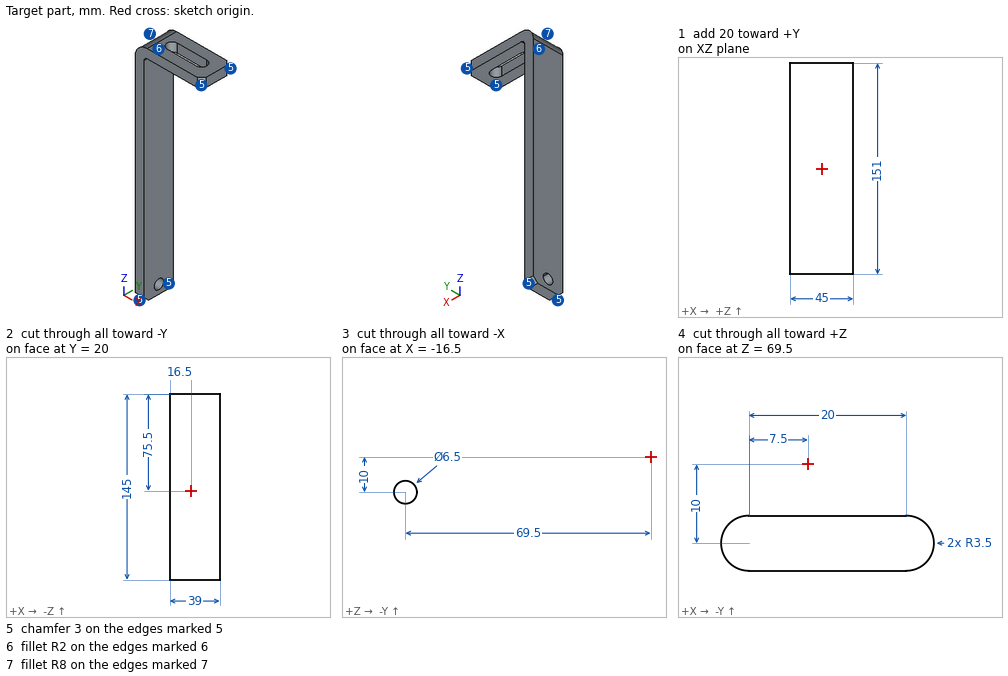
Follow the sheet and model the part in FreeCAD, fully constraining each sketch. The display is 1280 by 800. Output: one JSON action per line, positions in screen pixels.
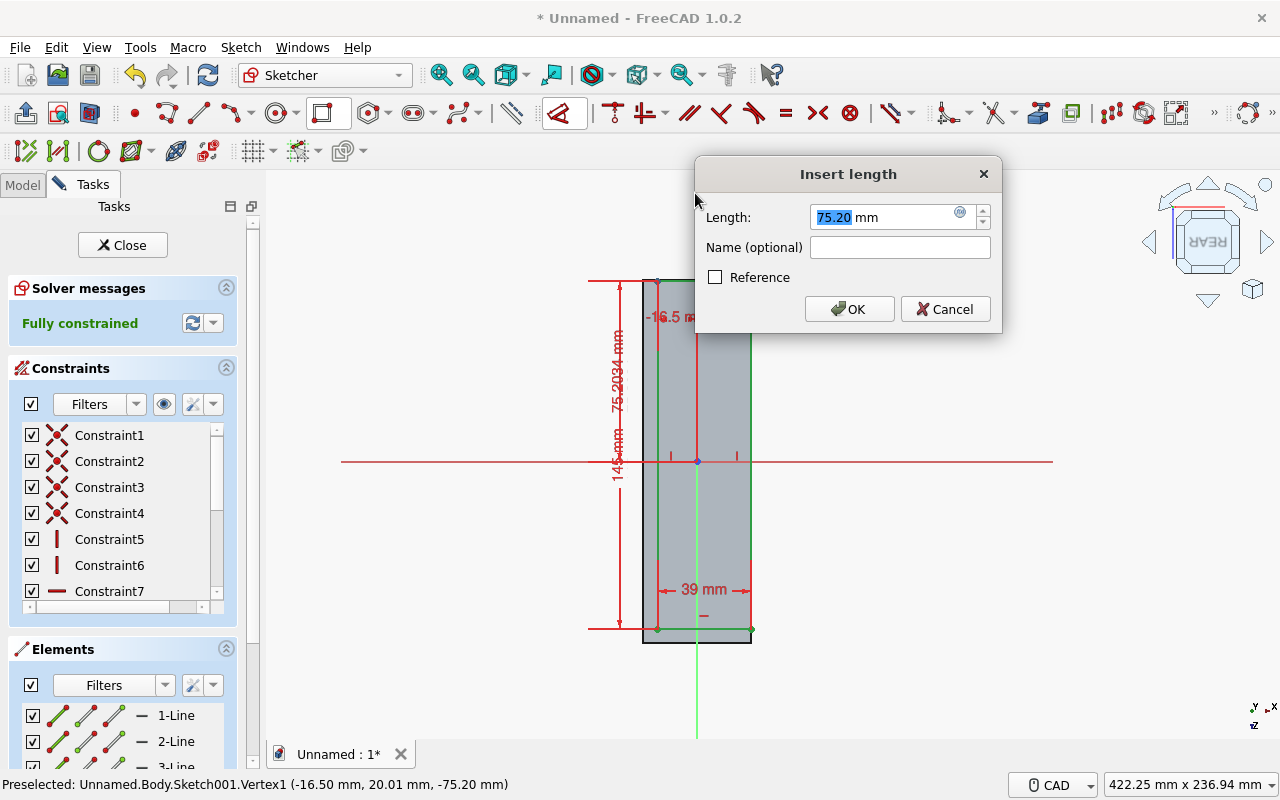
{"action": "type", "text": "75.5"}
{"action": "key", "text": "Return"}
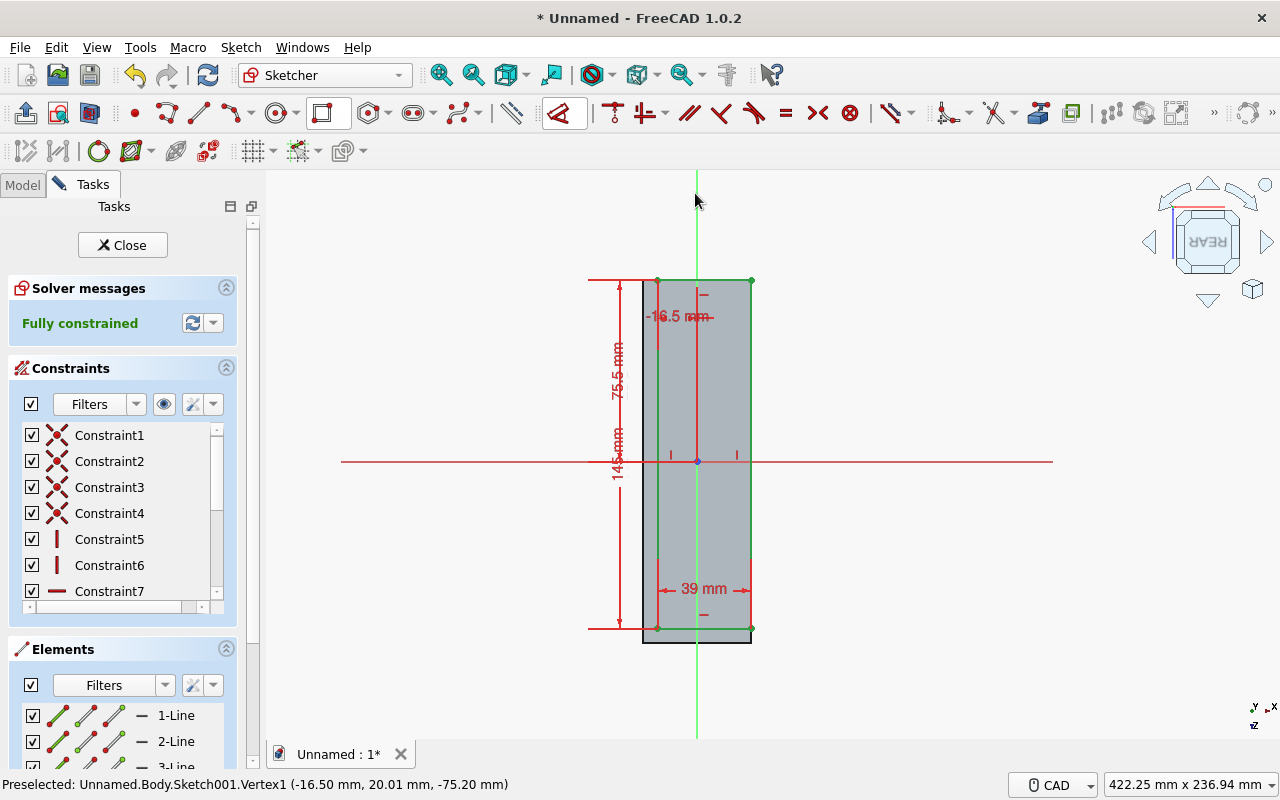
{"action": "left_click", "coordinate": [123, 245]}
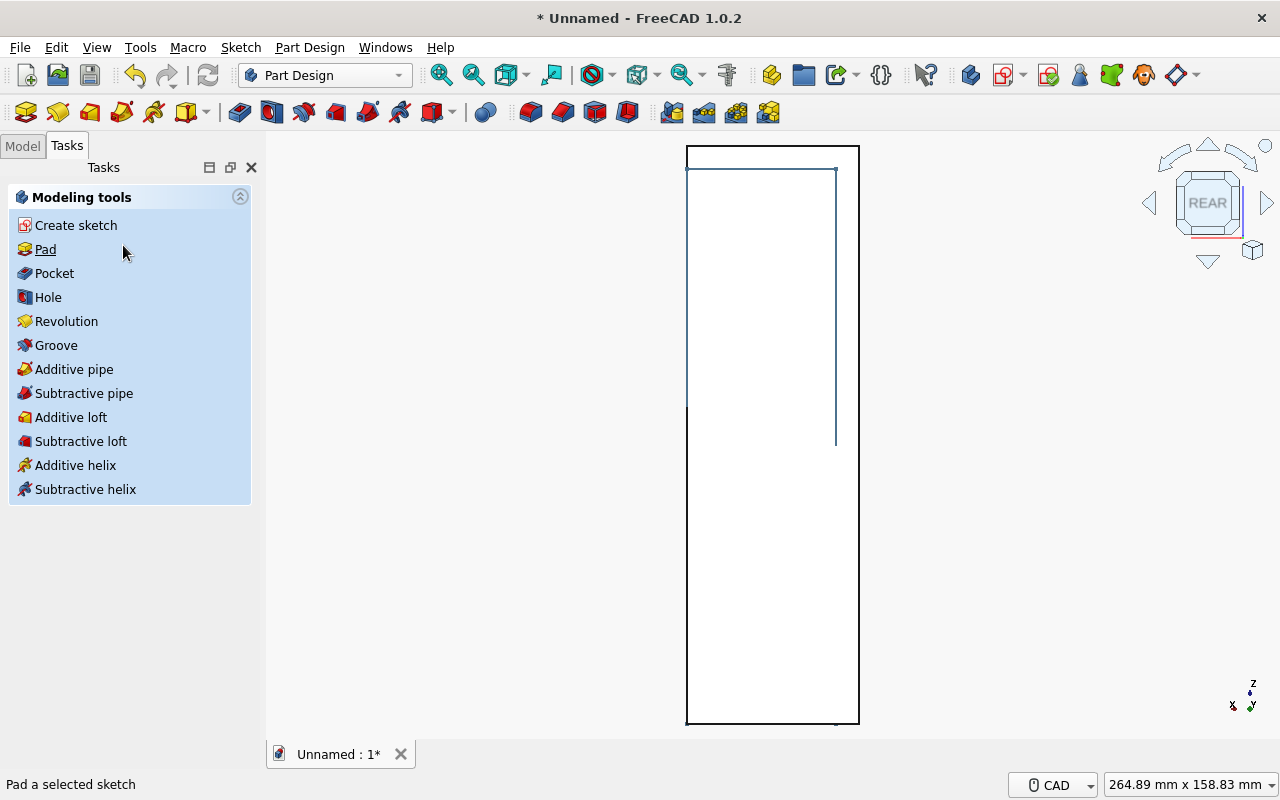
{"action": "left_click", "coordinate": [240, 112]}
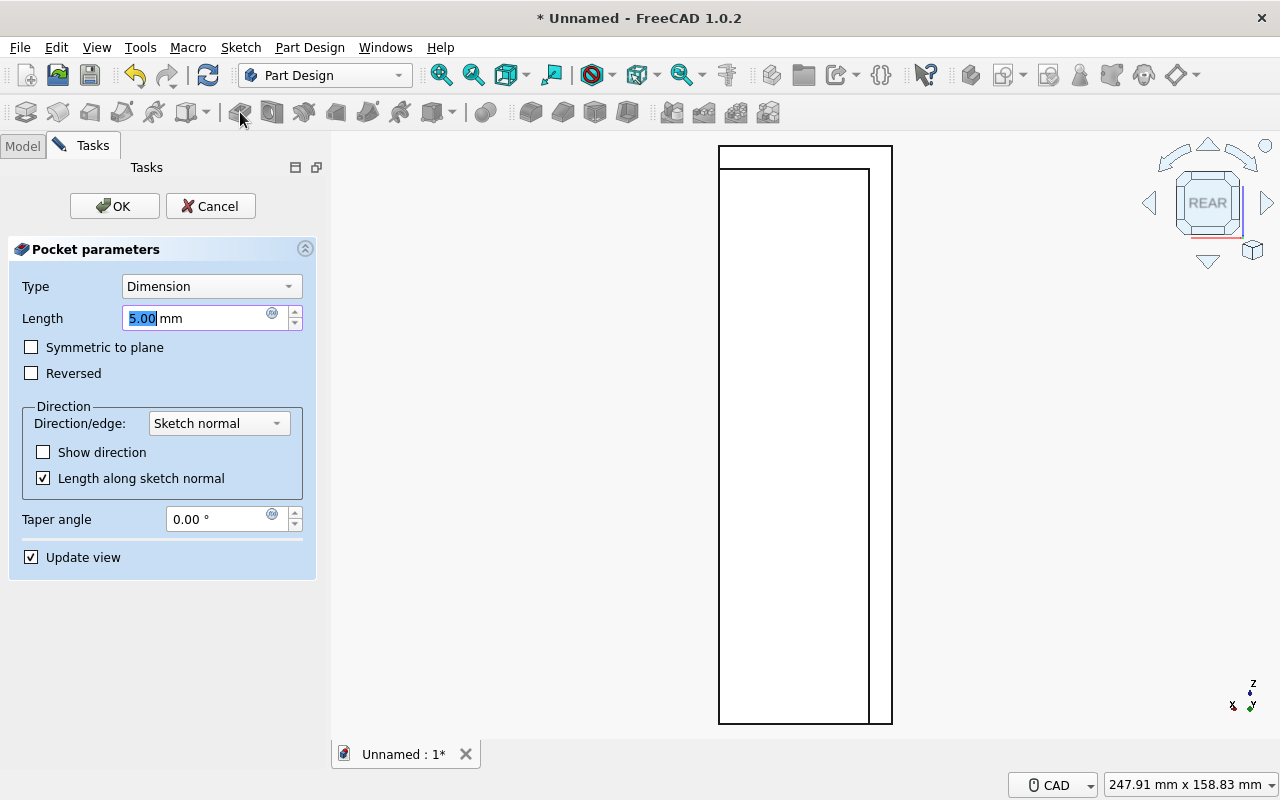
{"action": "left_click", "coordinate": [212, 286]}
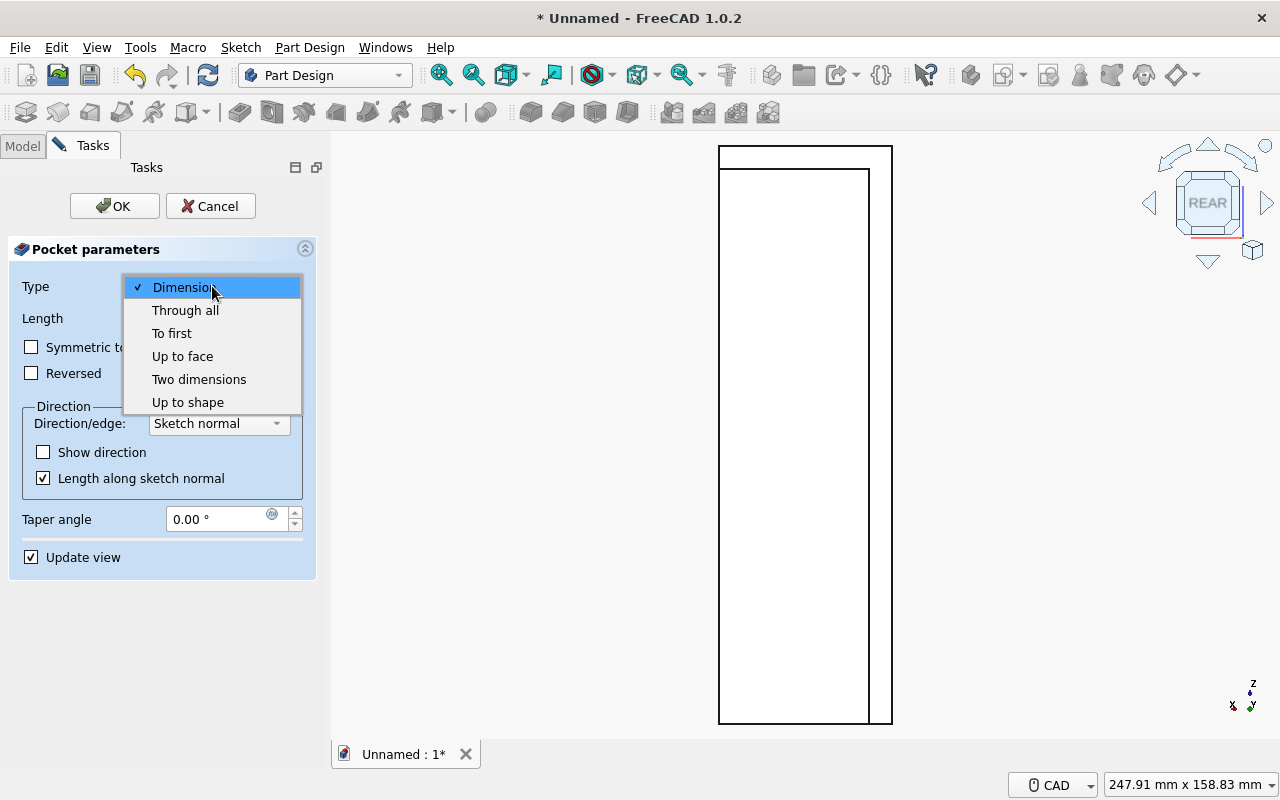
{"action": "left_click", "coordinate": [212, 310]}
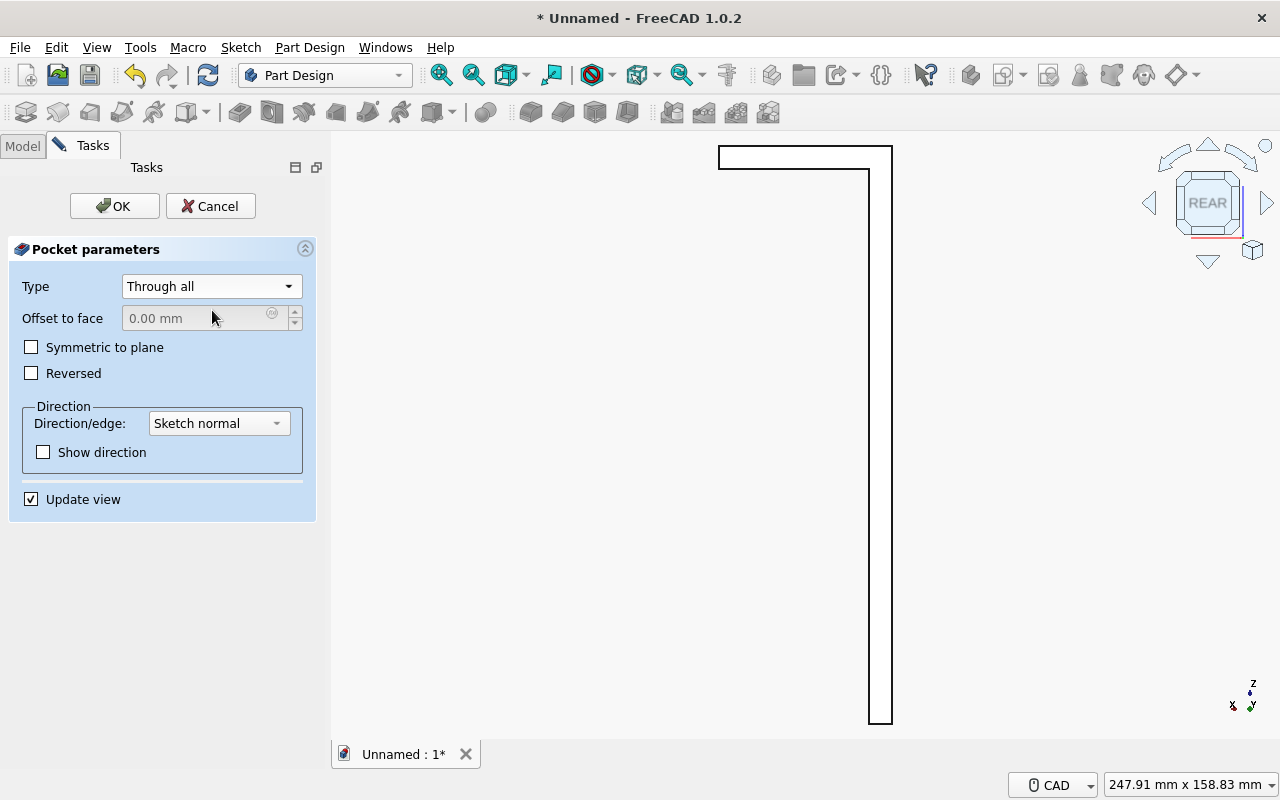
{"action": "left_click", "coordinate": [115, 206]}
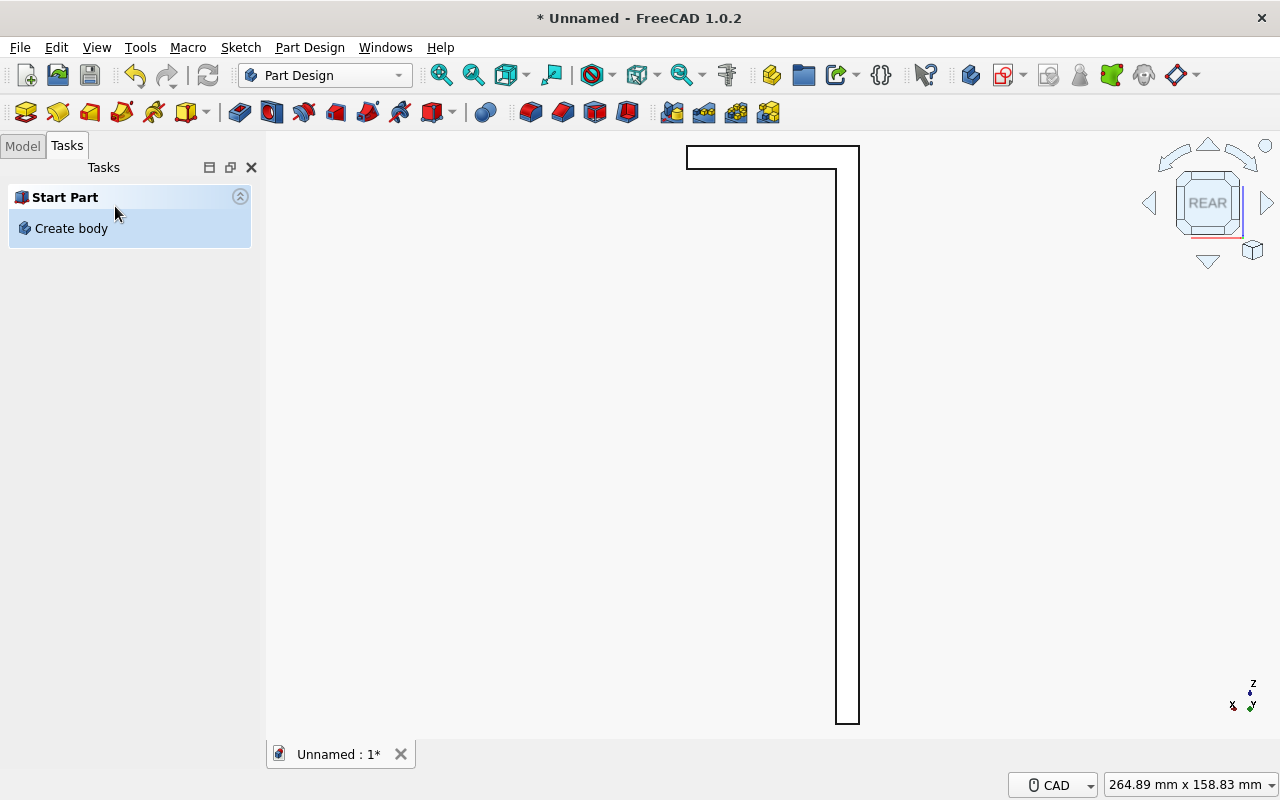
{"action": "key", "text": "0"}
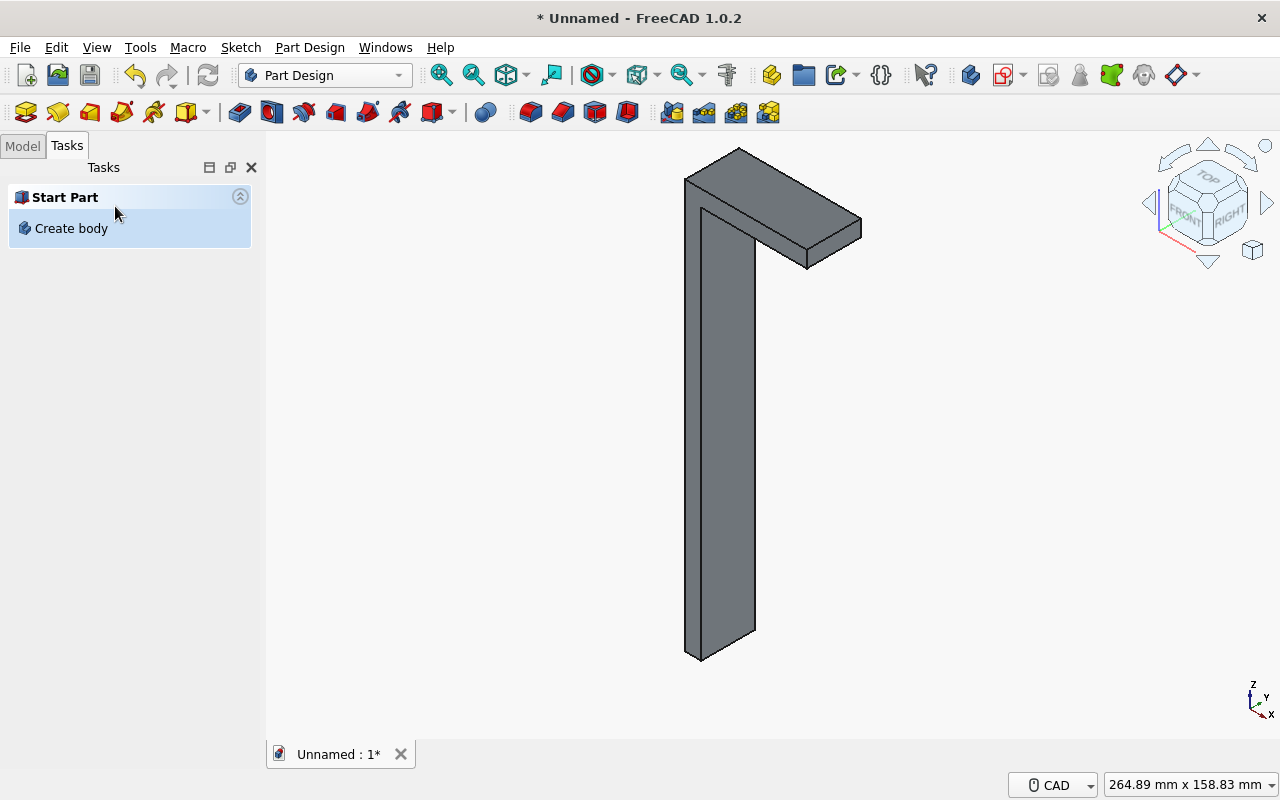
{"action": "left_click", "coordinate": [728, 612]}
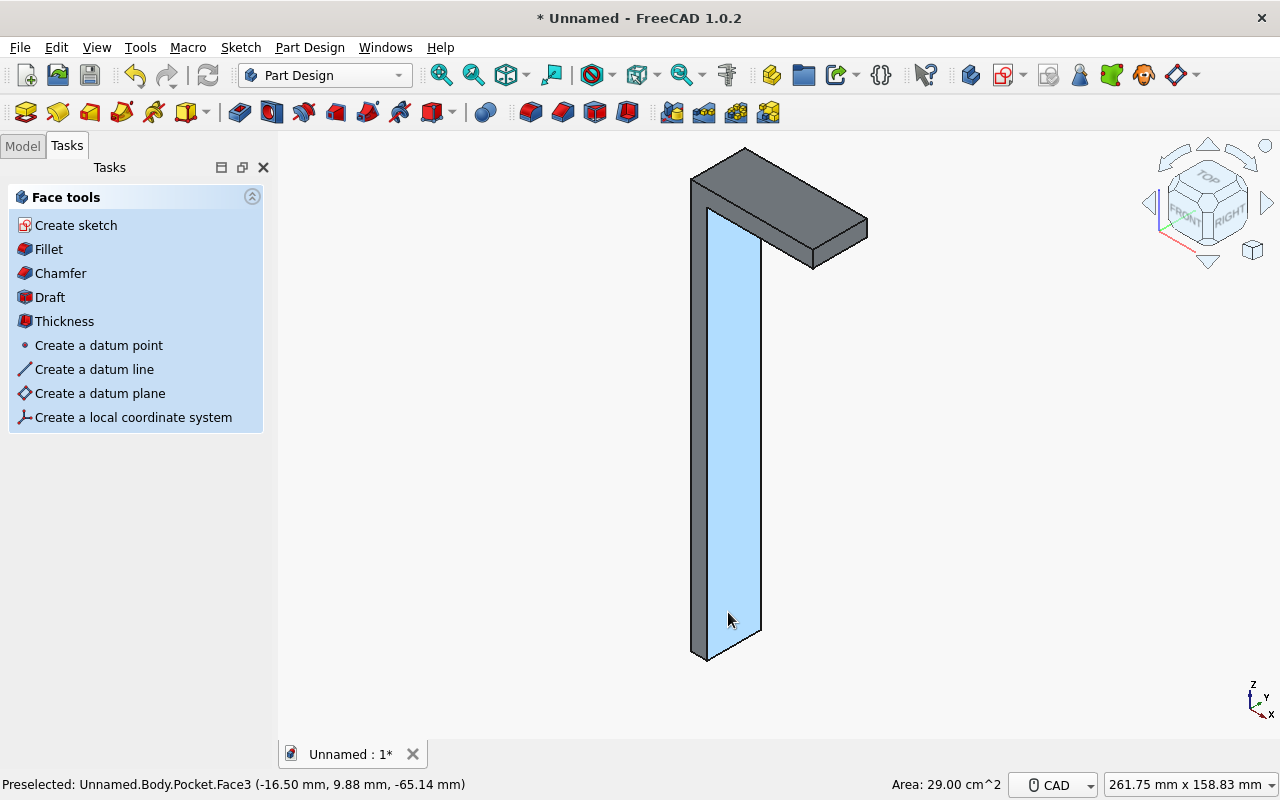
{"action": "left_click", "coordinate": [1004, 76]}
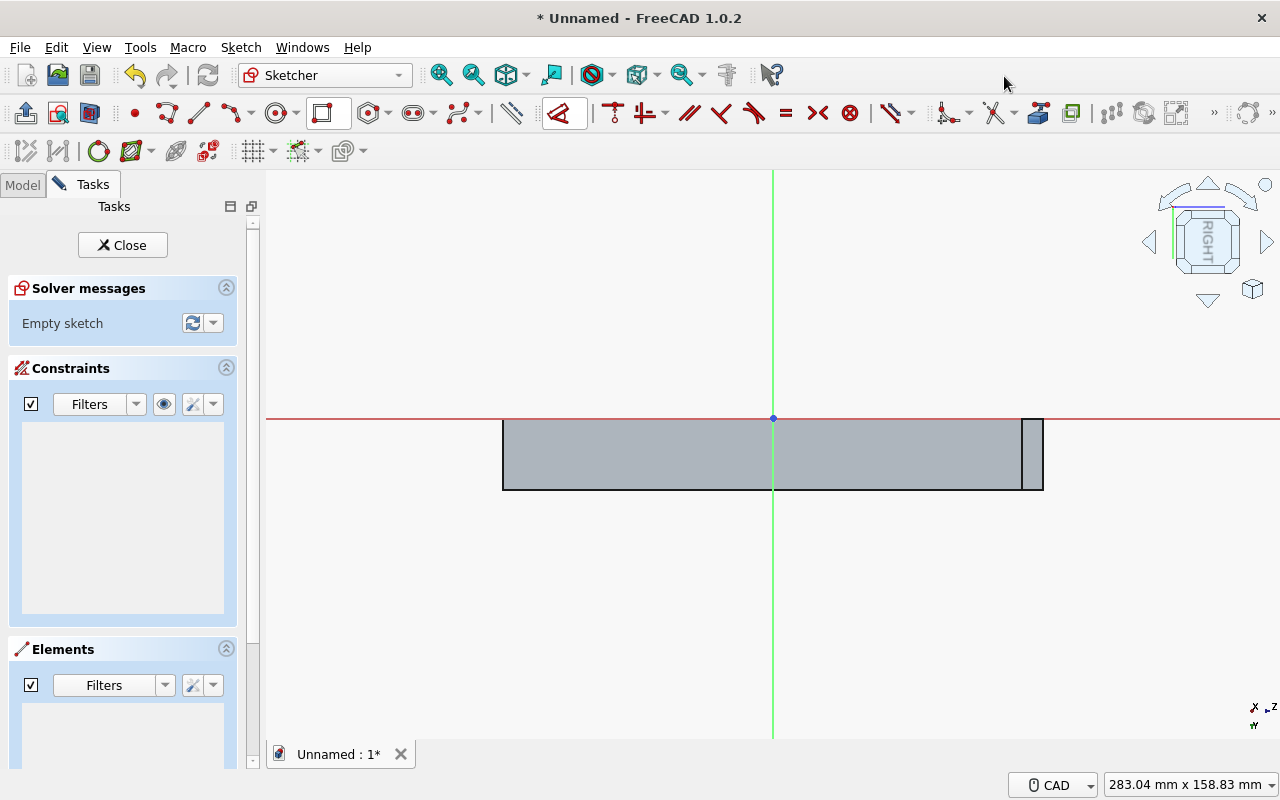
{"action": "scroll", "coordinate": [512, 455], "scroll_direction": "up", "scroll_amount": 14}